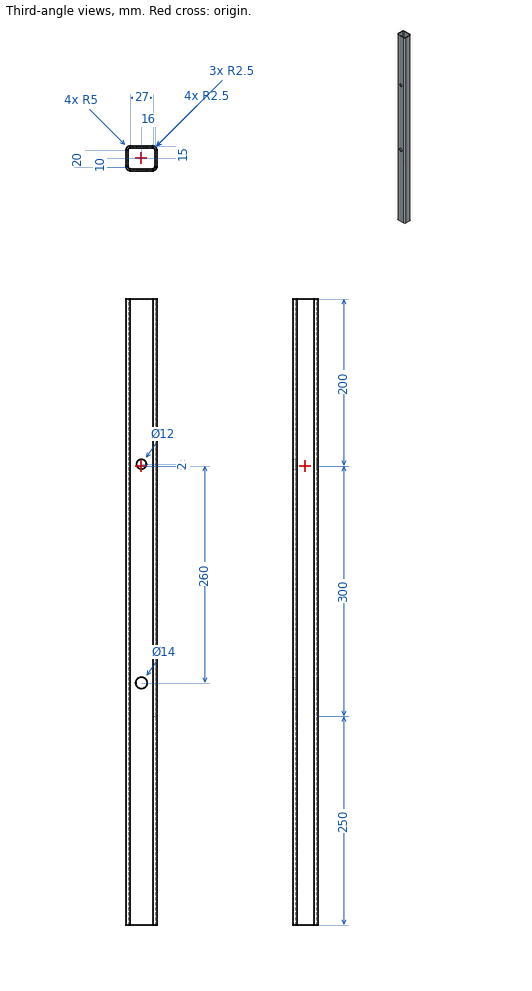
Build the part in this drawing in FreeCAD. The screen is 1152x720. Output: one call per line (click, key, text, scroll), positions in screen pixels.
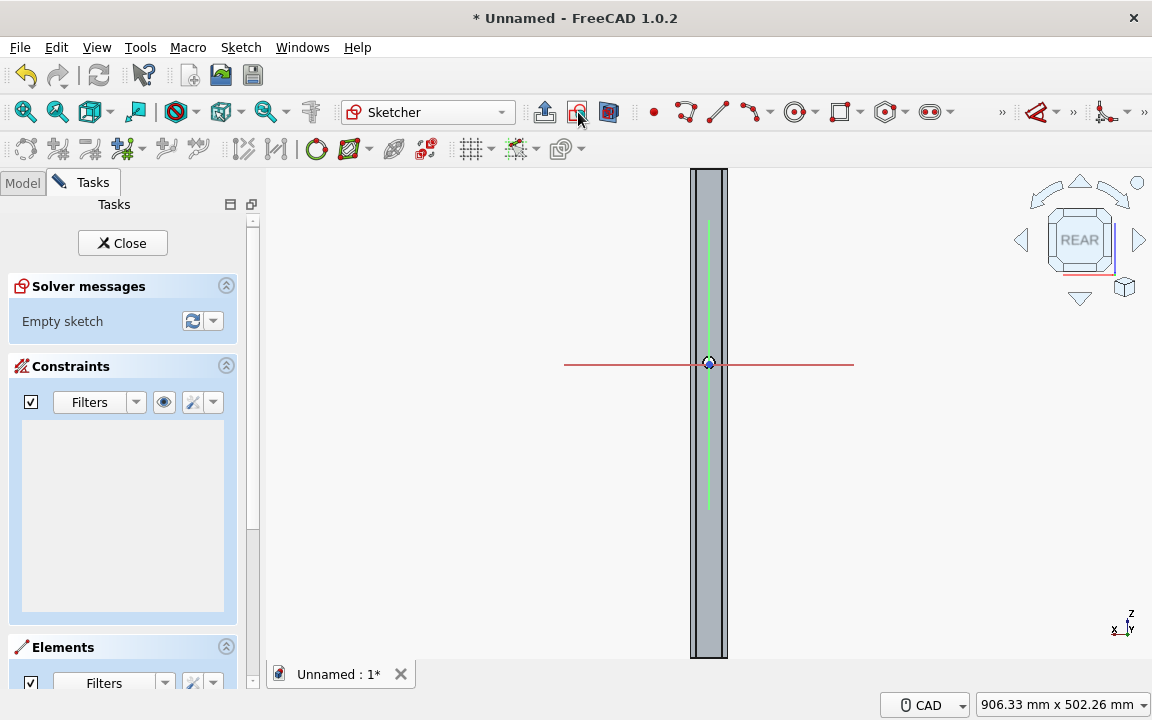
scroll(713, 630, up, 15)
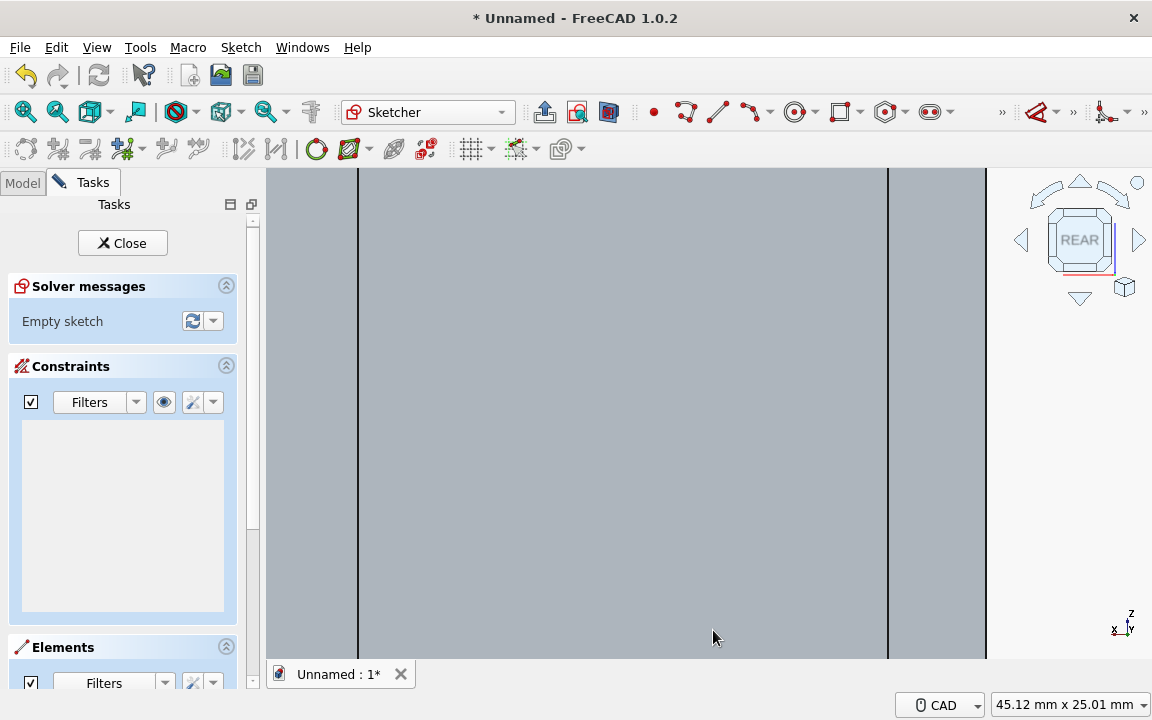
key(g)
key(c)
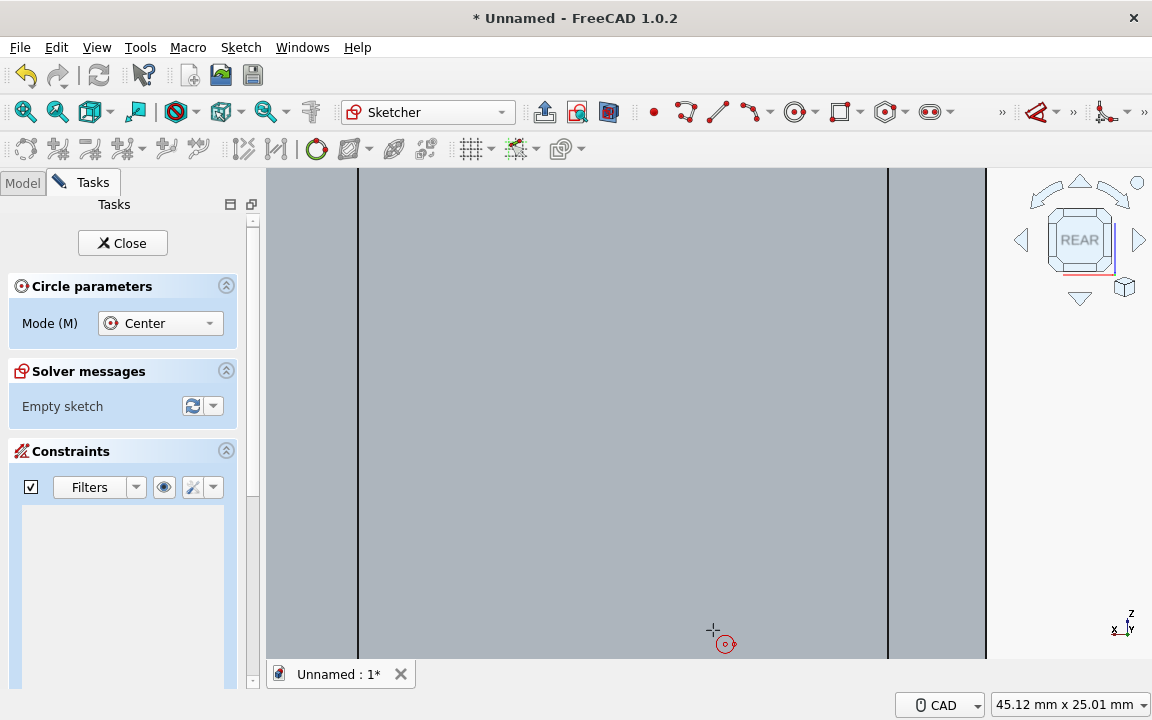
click(623, 387)
click(720, 290)
key(Escape)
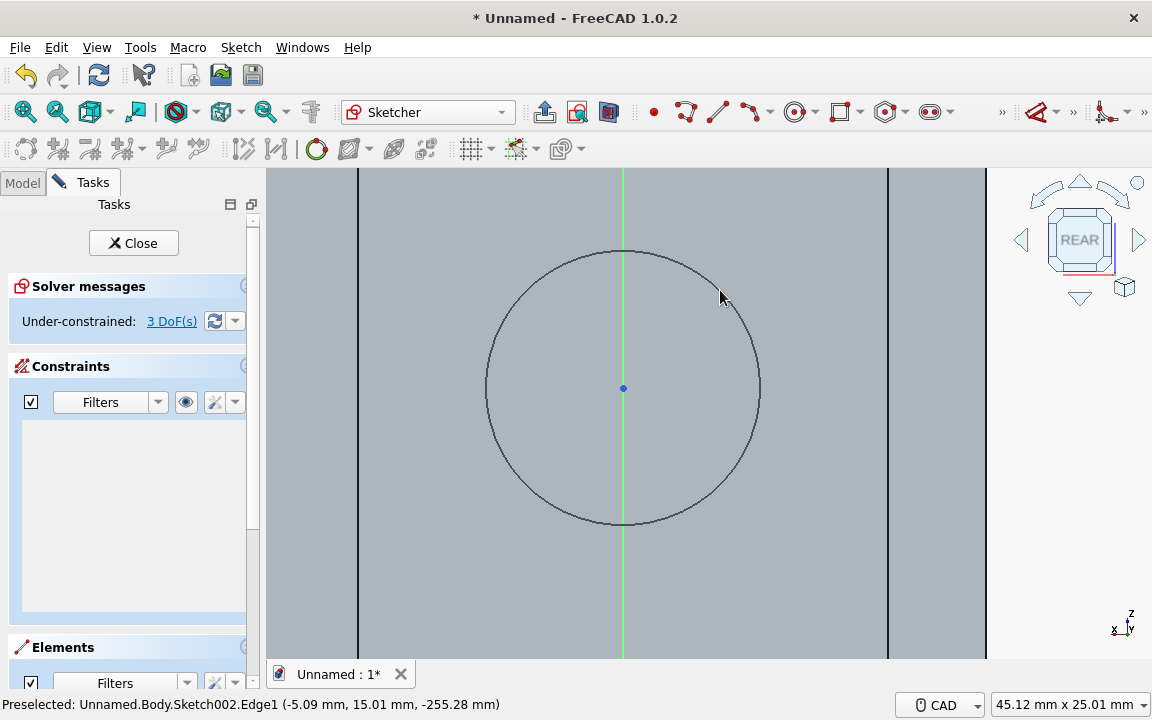
click(623, 388)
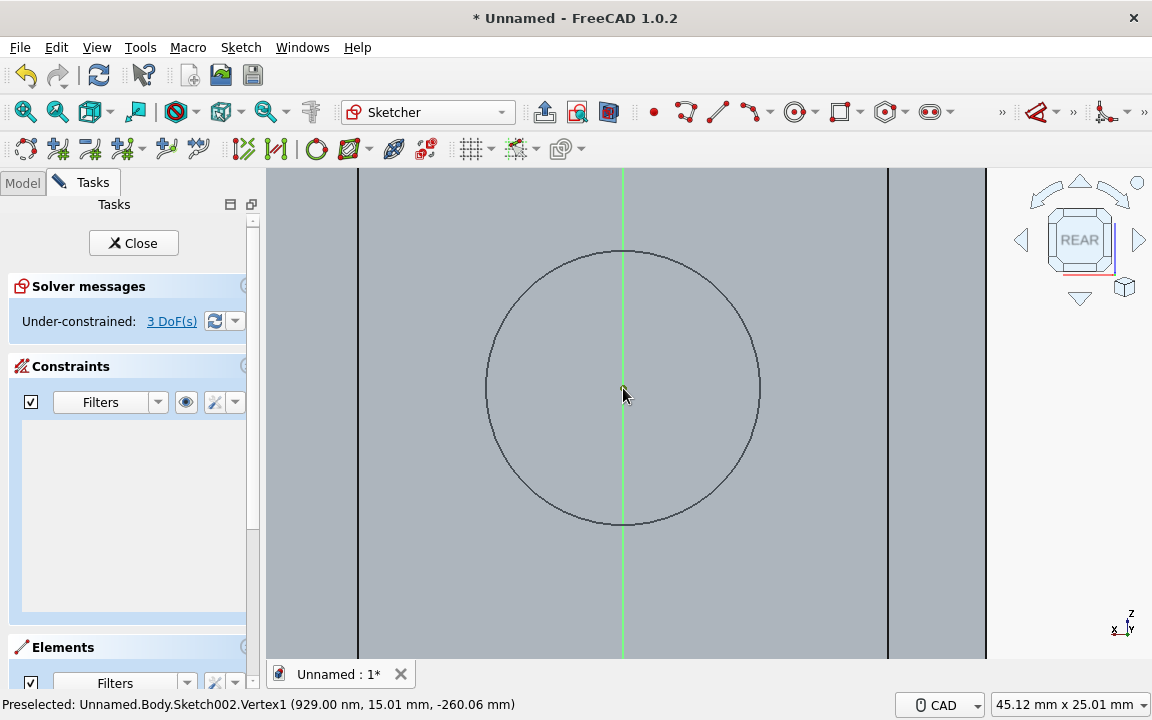
click(623, 600)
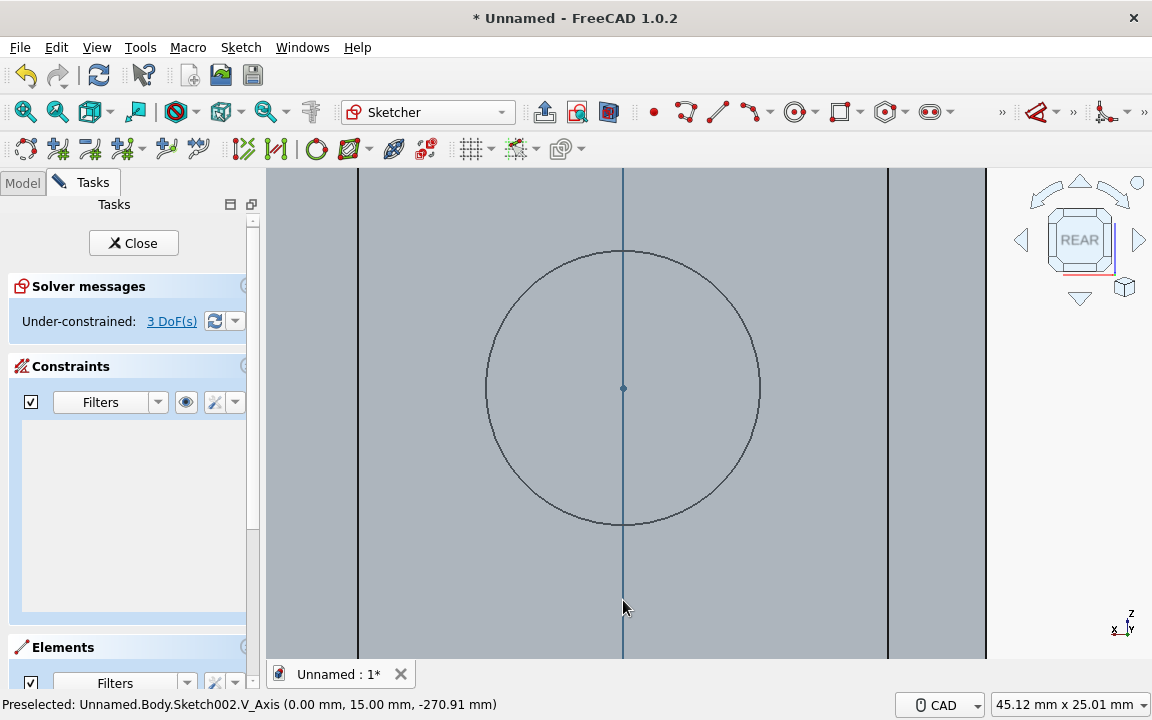
key(c)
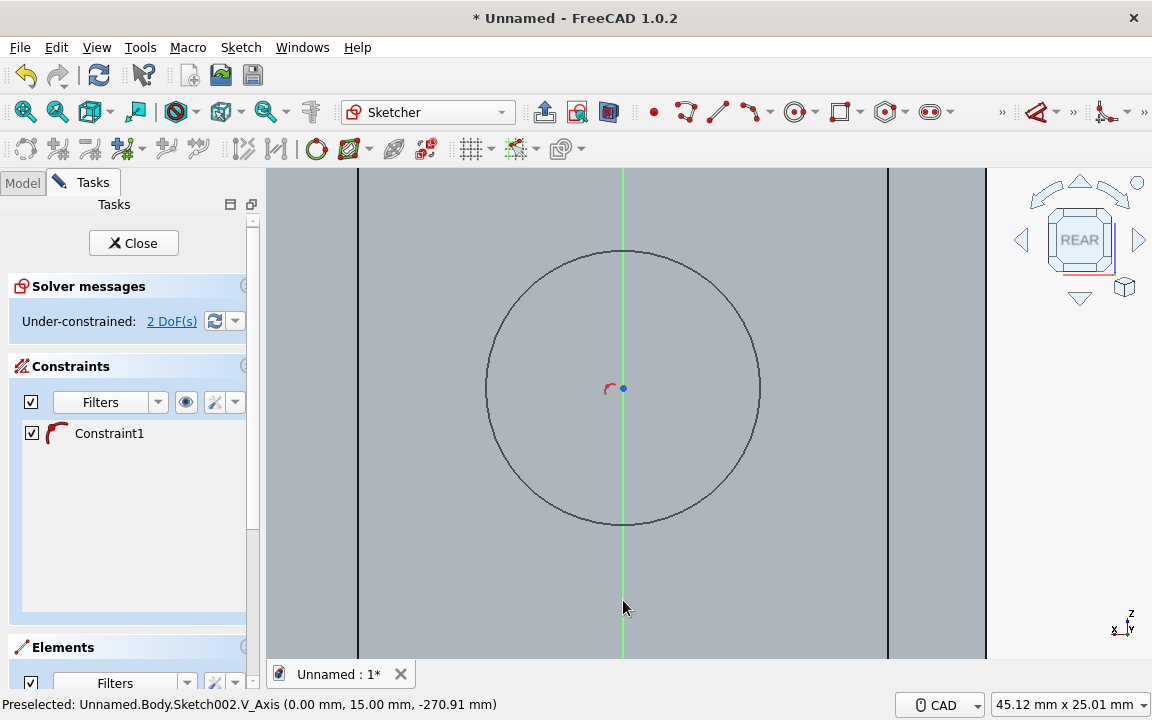
key(d)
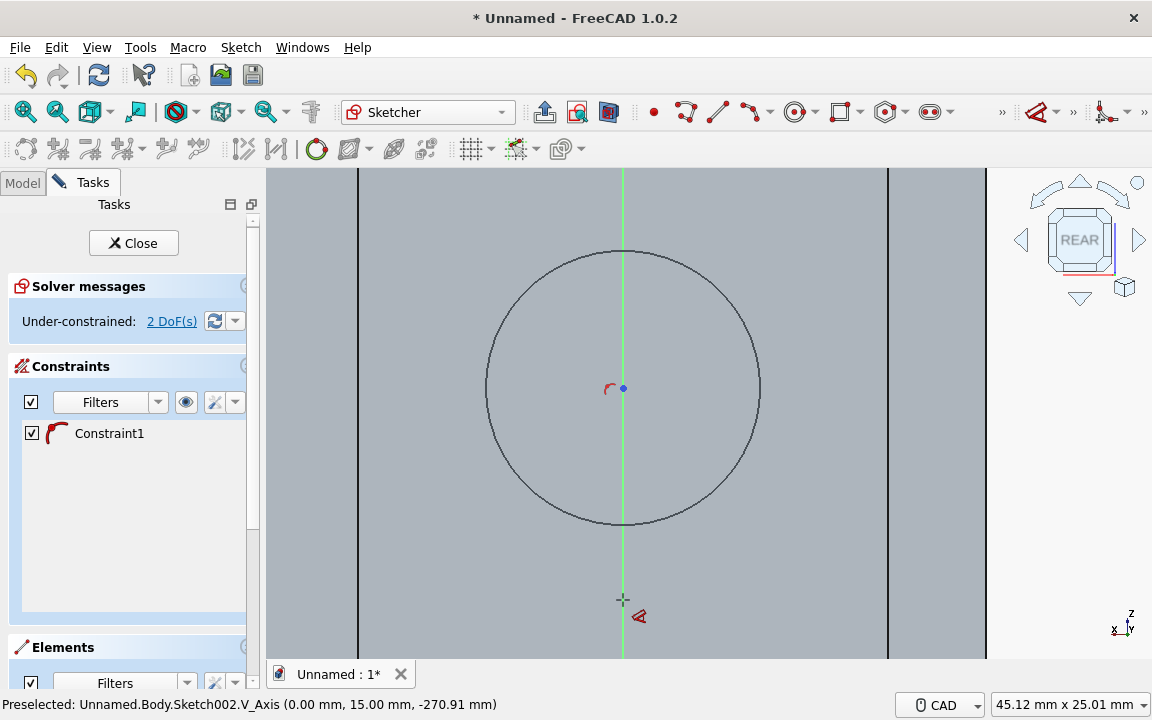
click(720, 291)
click(743, 268)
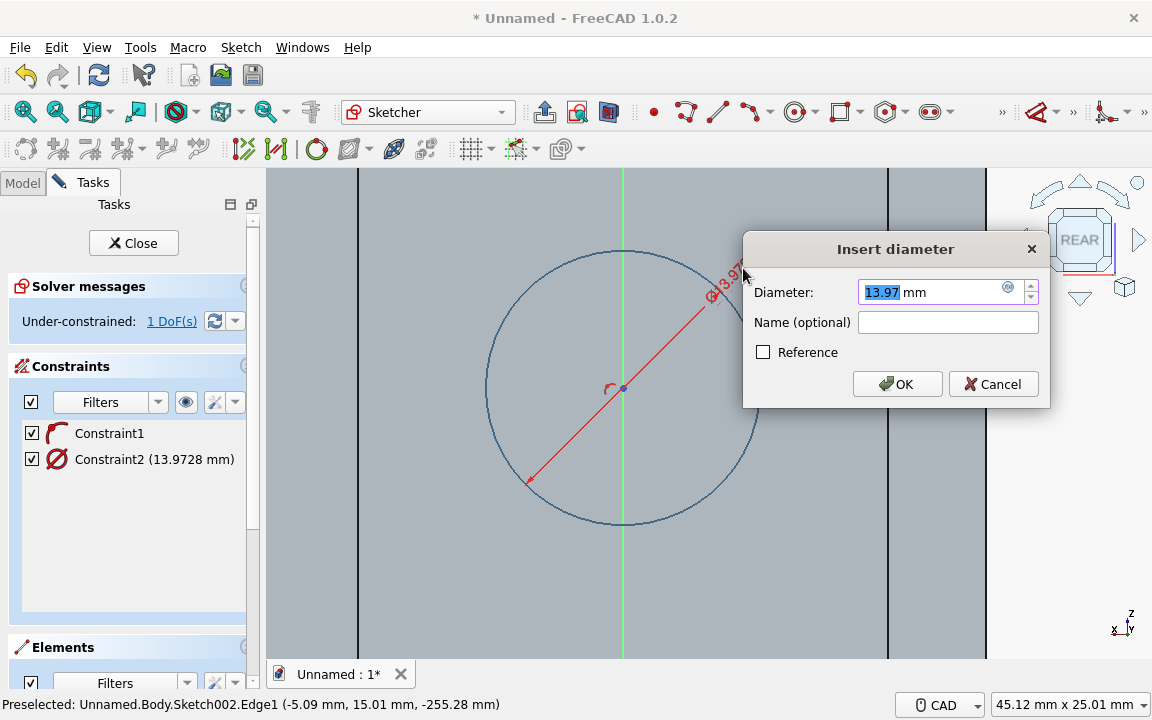
text(14)
key(Return)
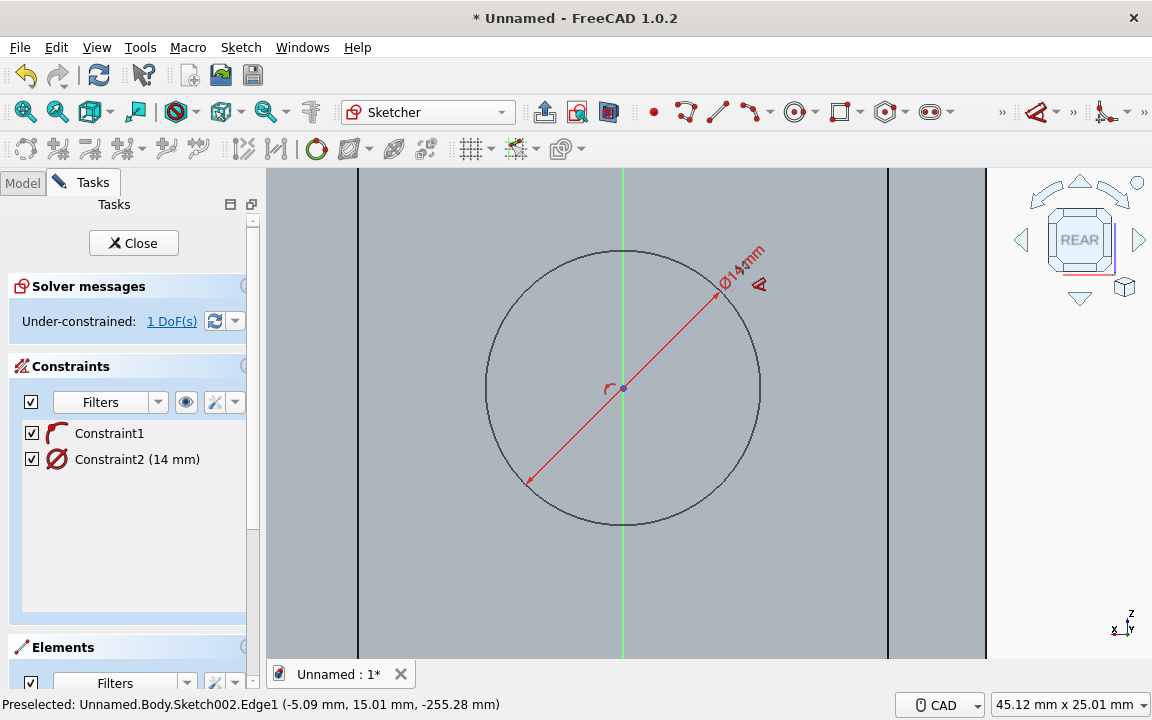
click(623, 388)
click(657, 292)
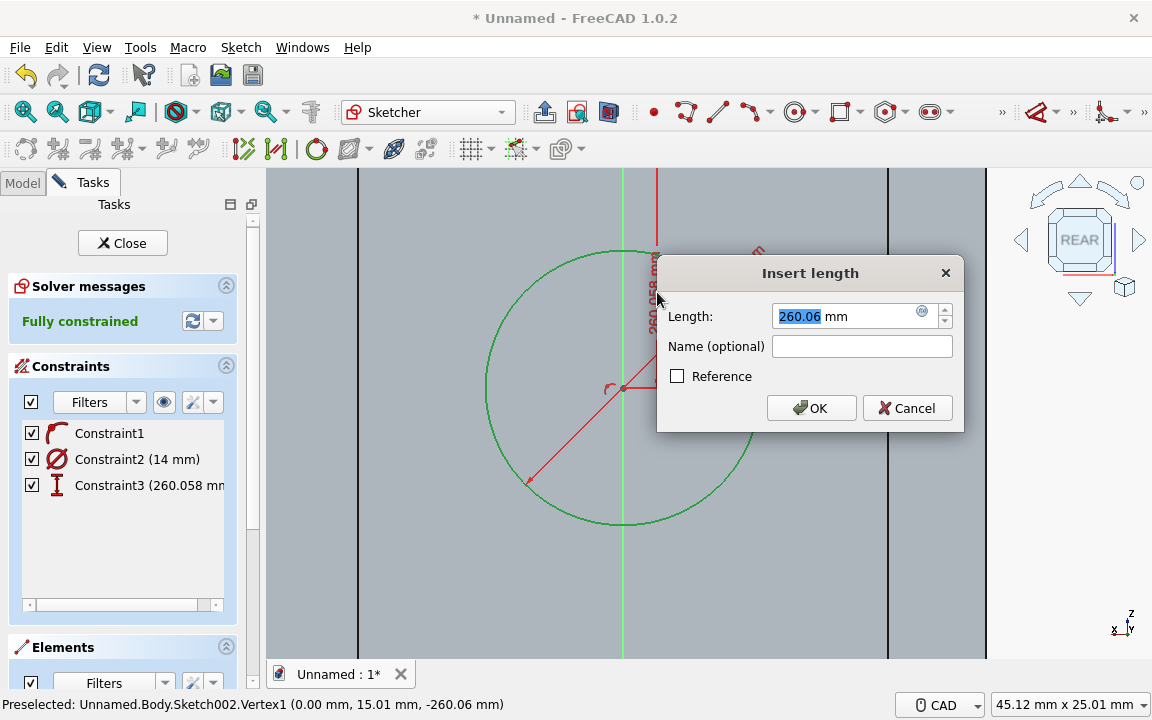
text(260)
key(Return)
key(Escape)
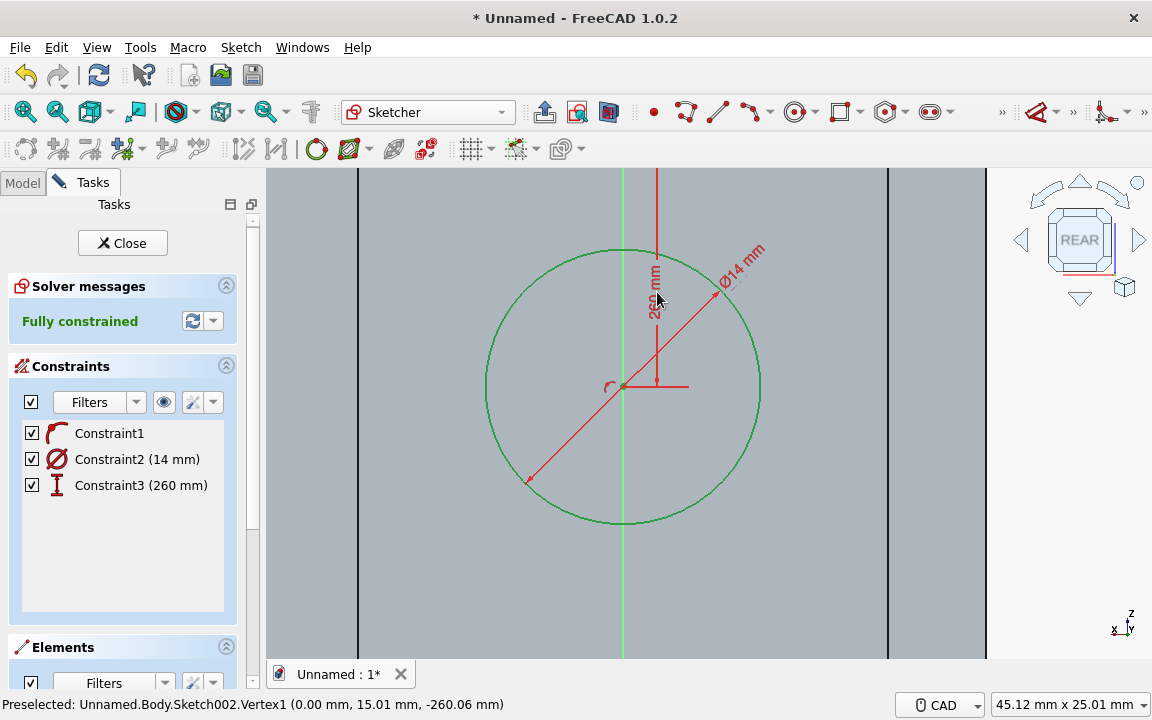
click(123, 243)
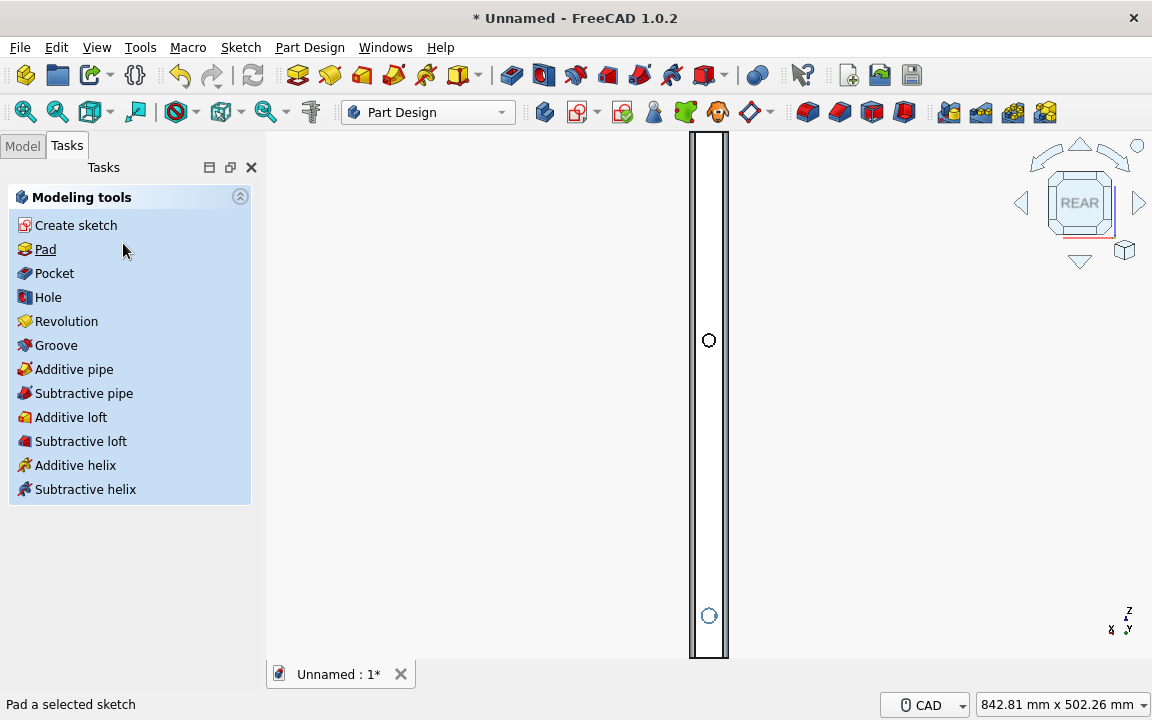
click(512, 76)